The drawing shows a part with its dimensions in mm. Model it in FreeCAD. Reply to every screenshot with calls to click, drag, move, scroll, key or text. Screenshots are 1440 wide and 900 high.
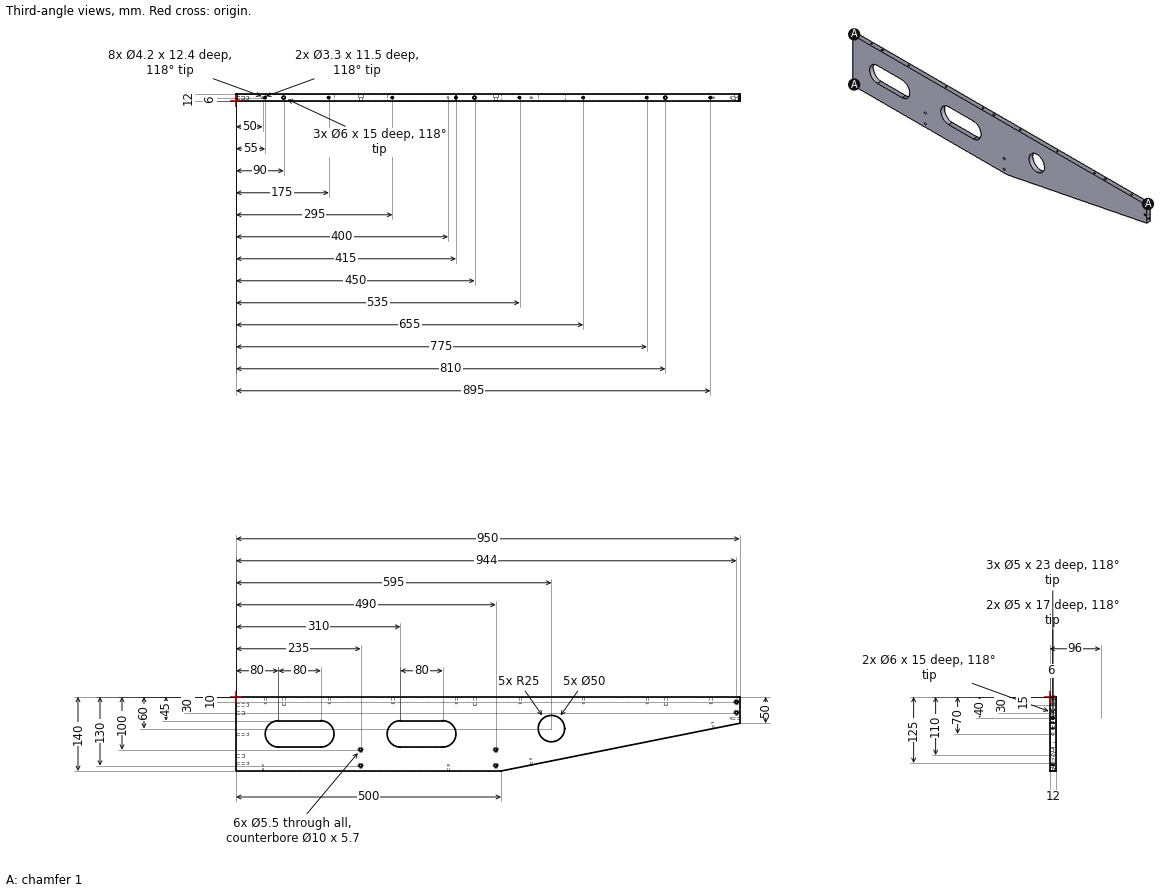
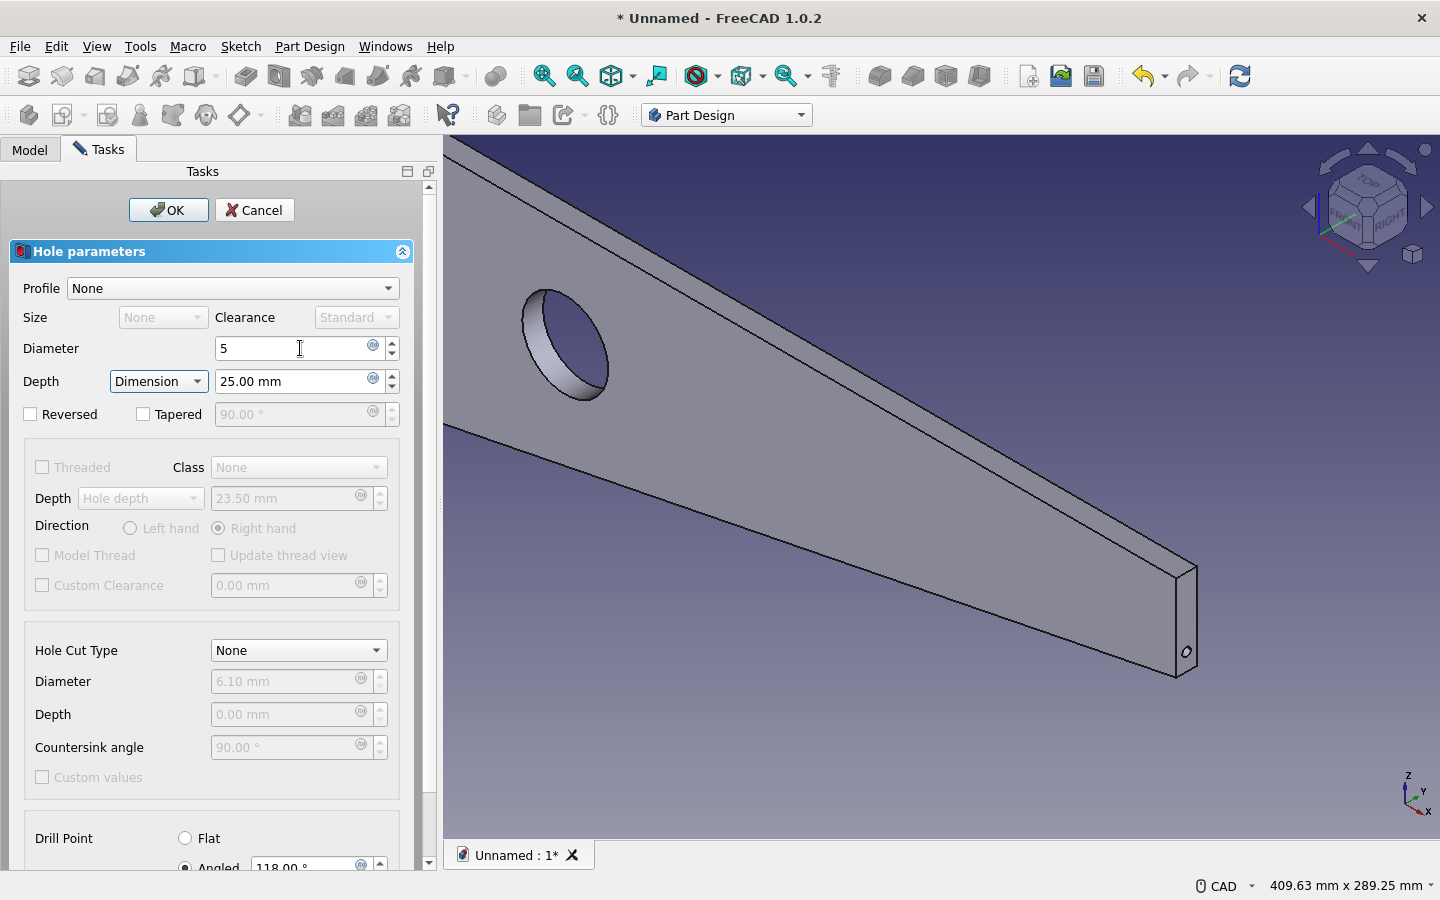
triple_click(300, 382)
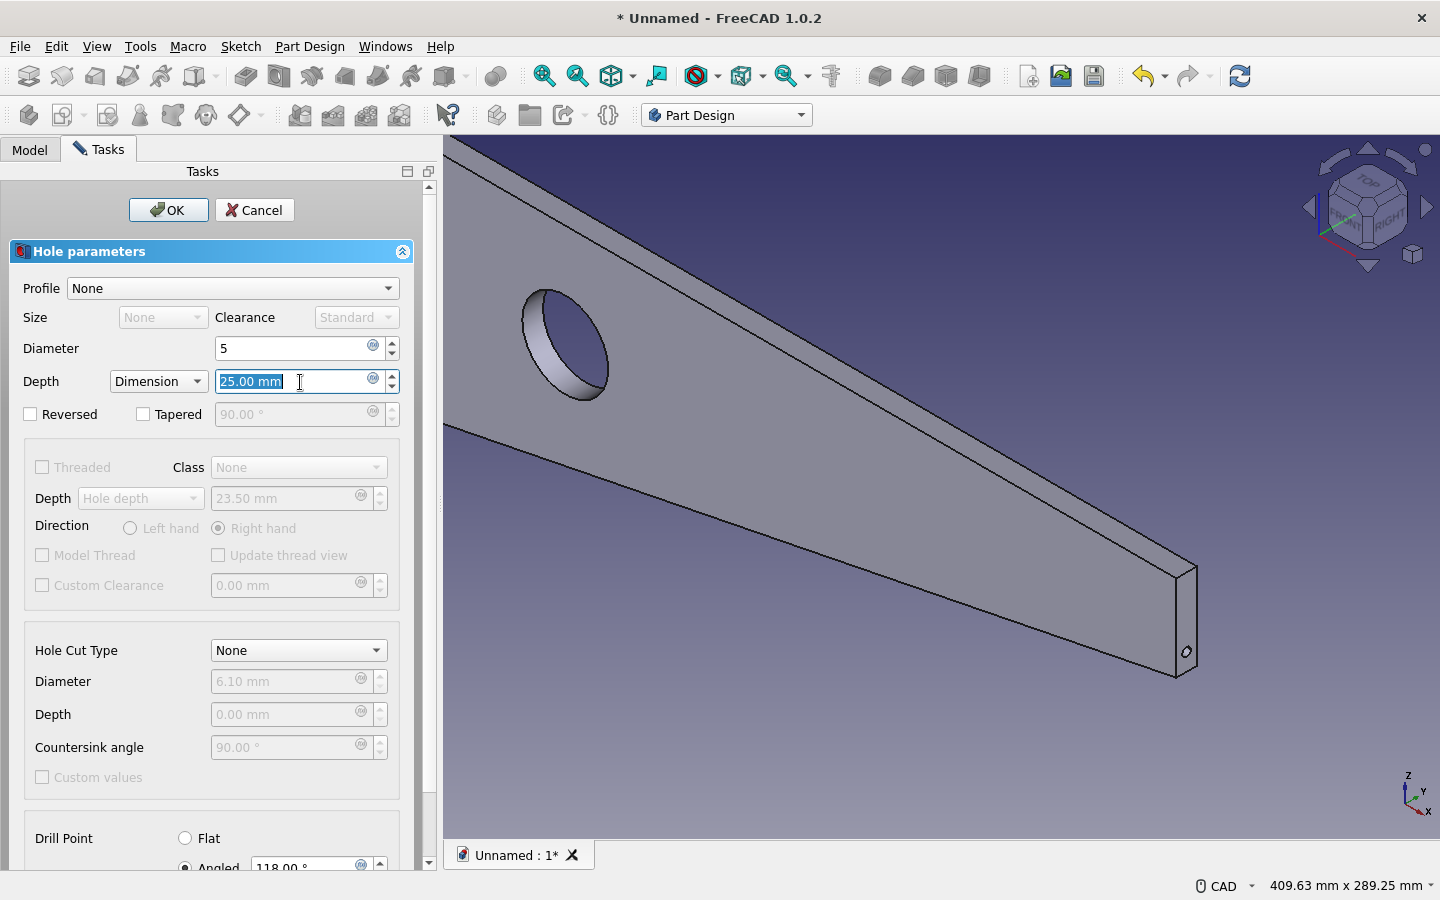
text(17)
key(Tab)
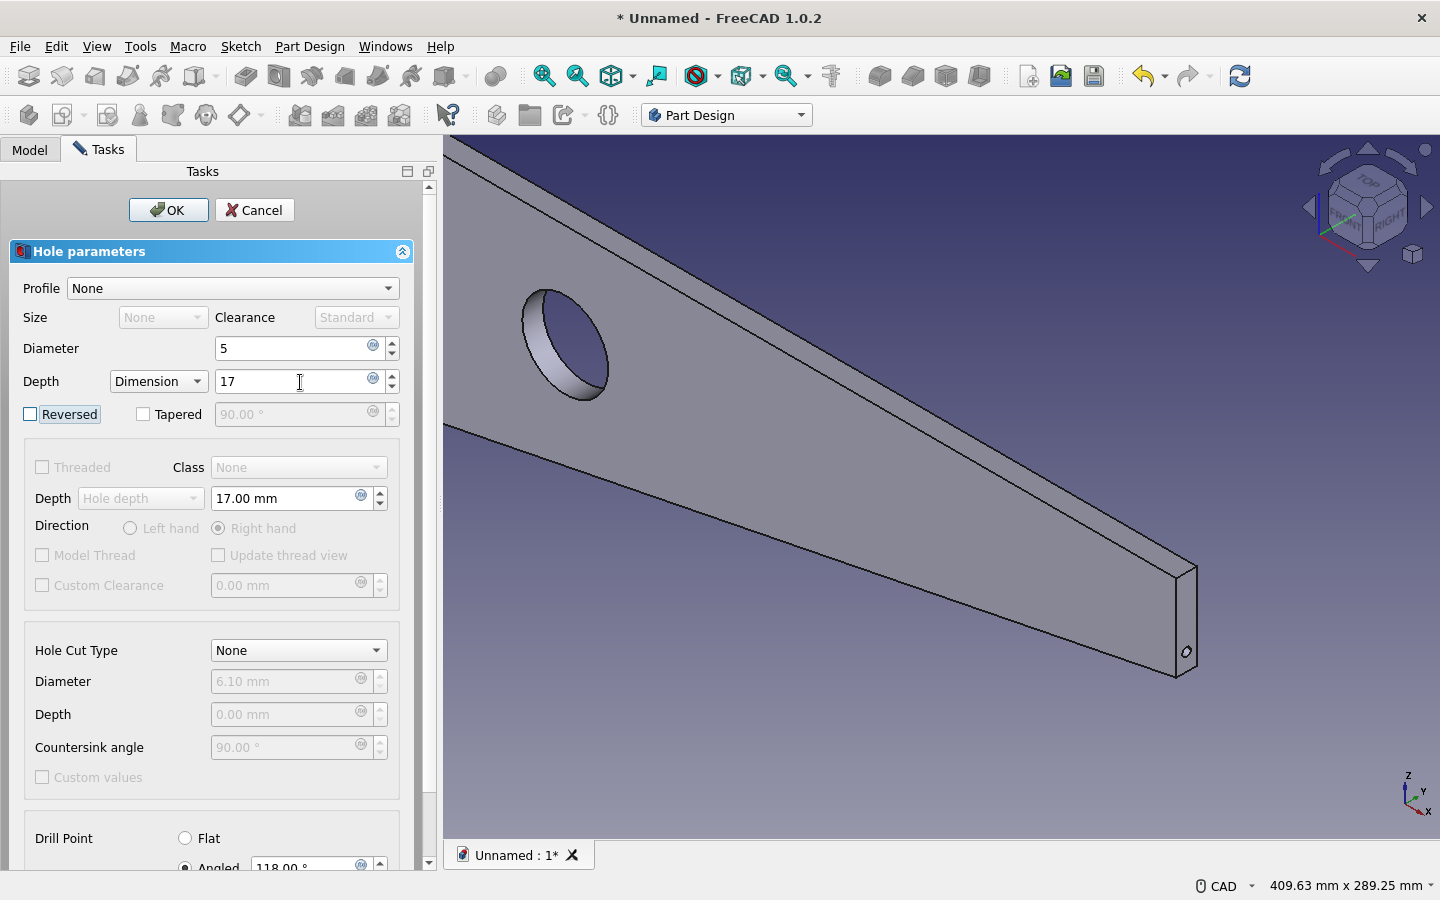
click(169, 210)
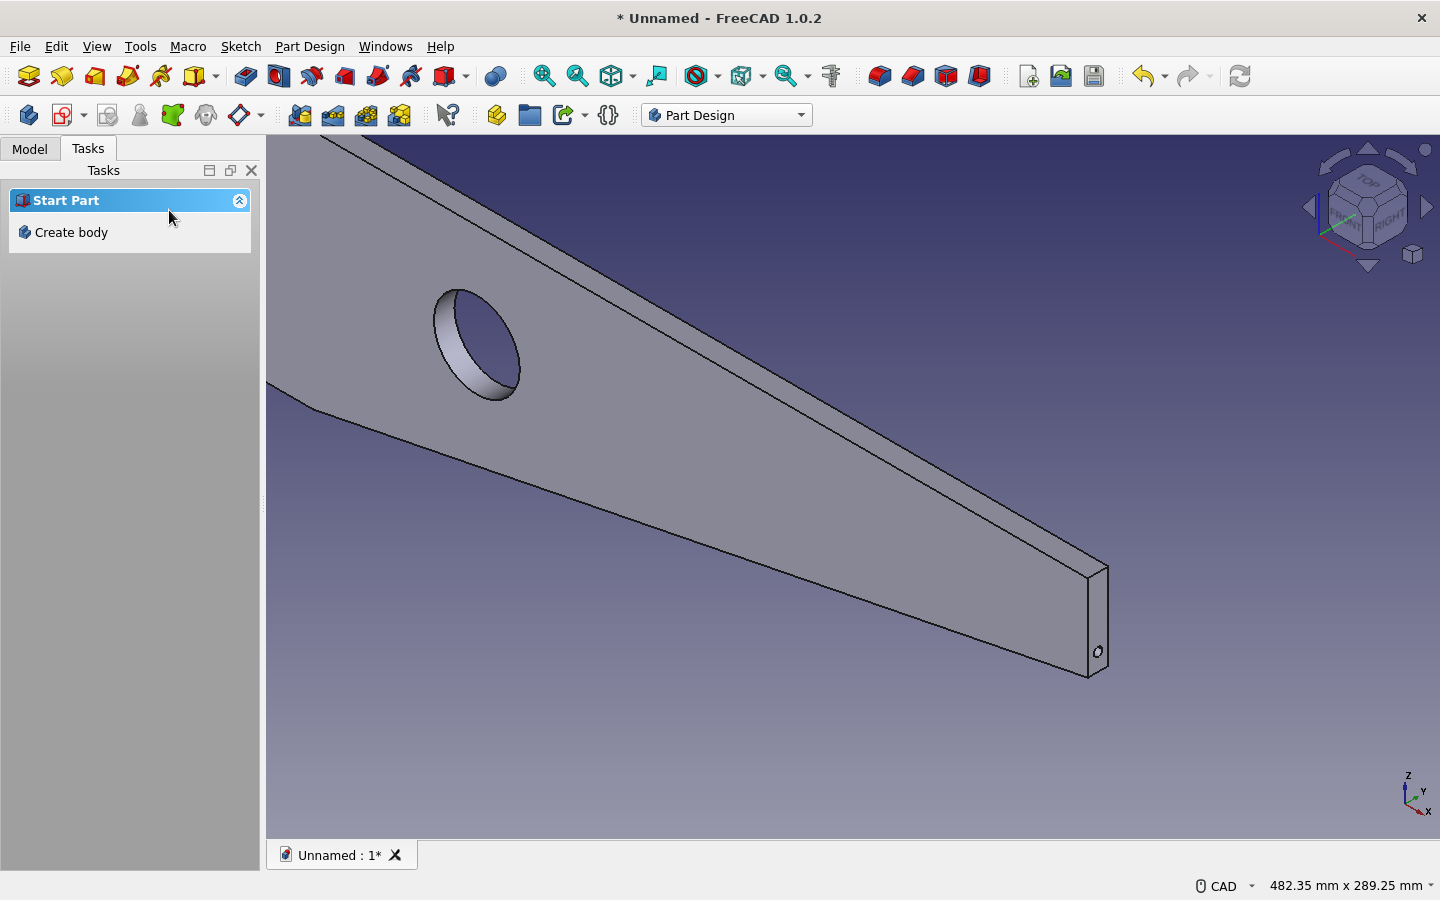
click(545, 76)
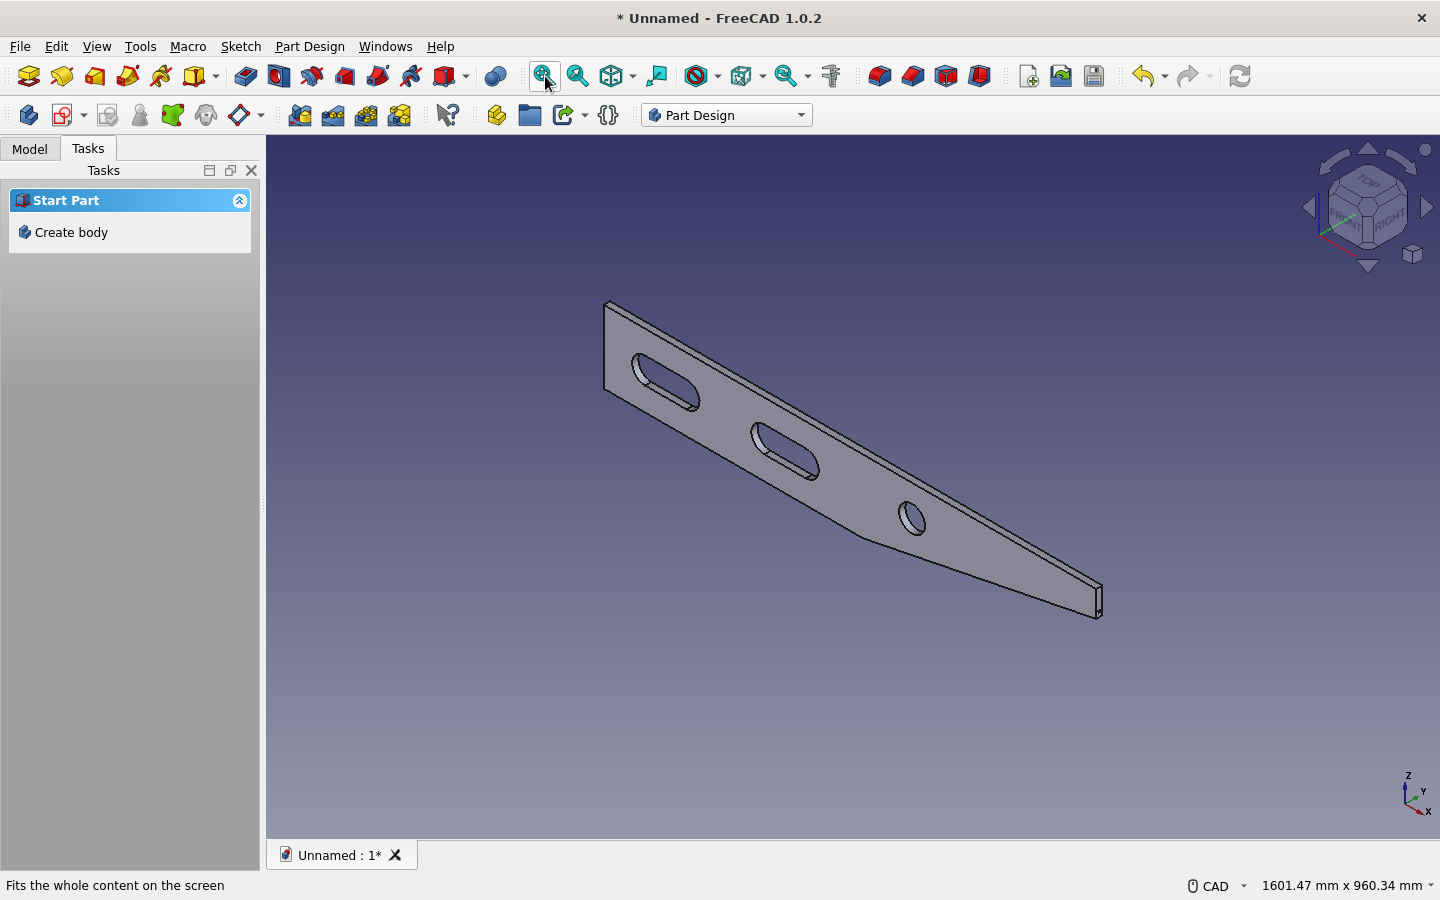
click(62, 116)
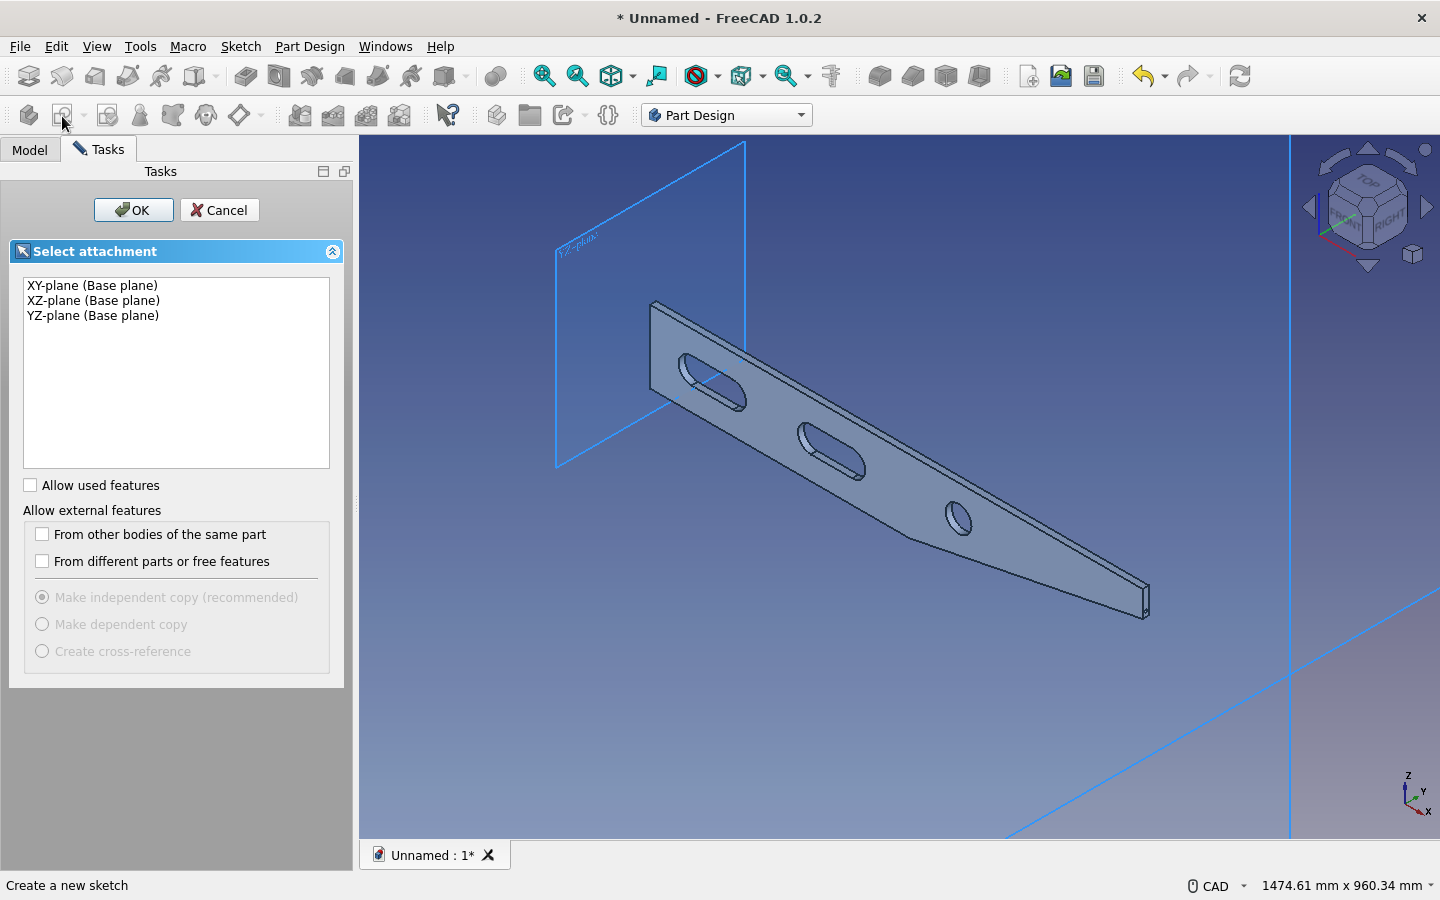
click(84, 316)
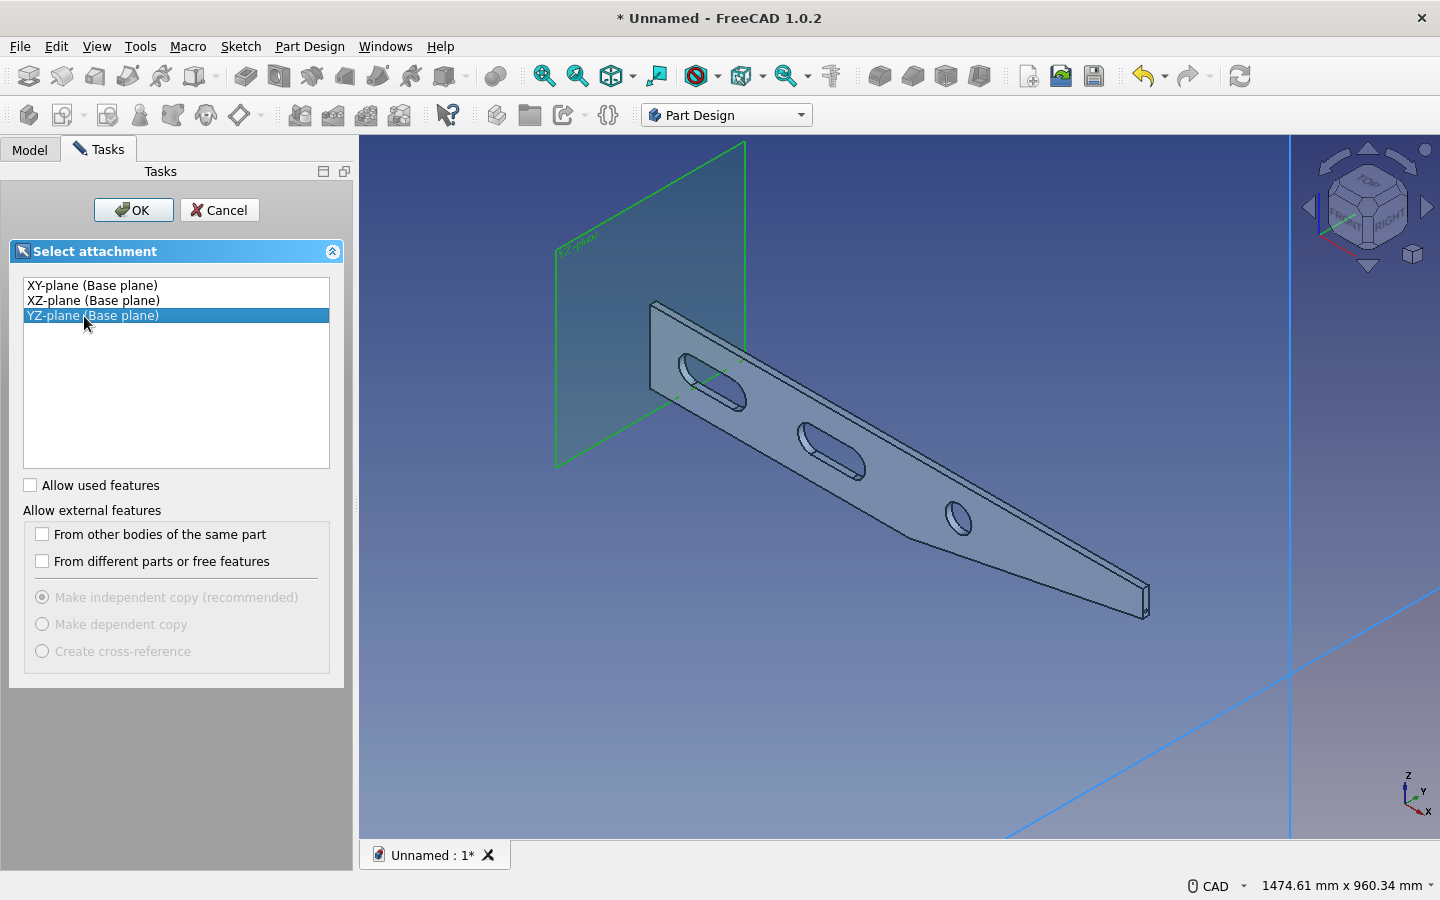
click(134, 210)